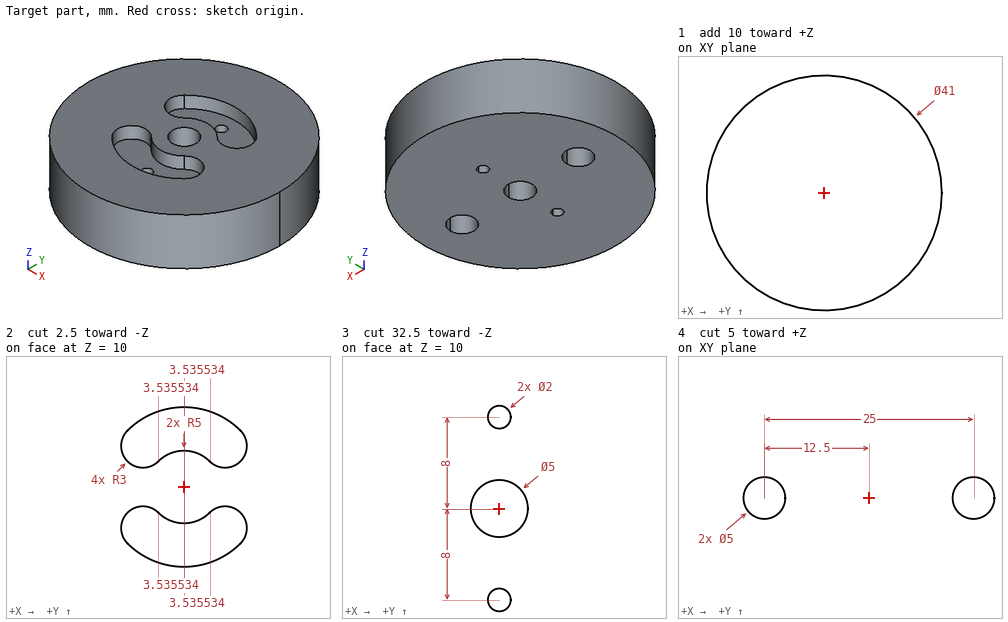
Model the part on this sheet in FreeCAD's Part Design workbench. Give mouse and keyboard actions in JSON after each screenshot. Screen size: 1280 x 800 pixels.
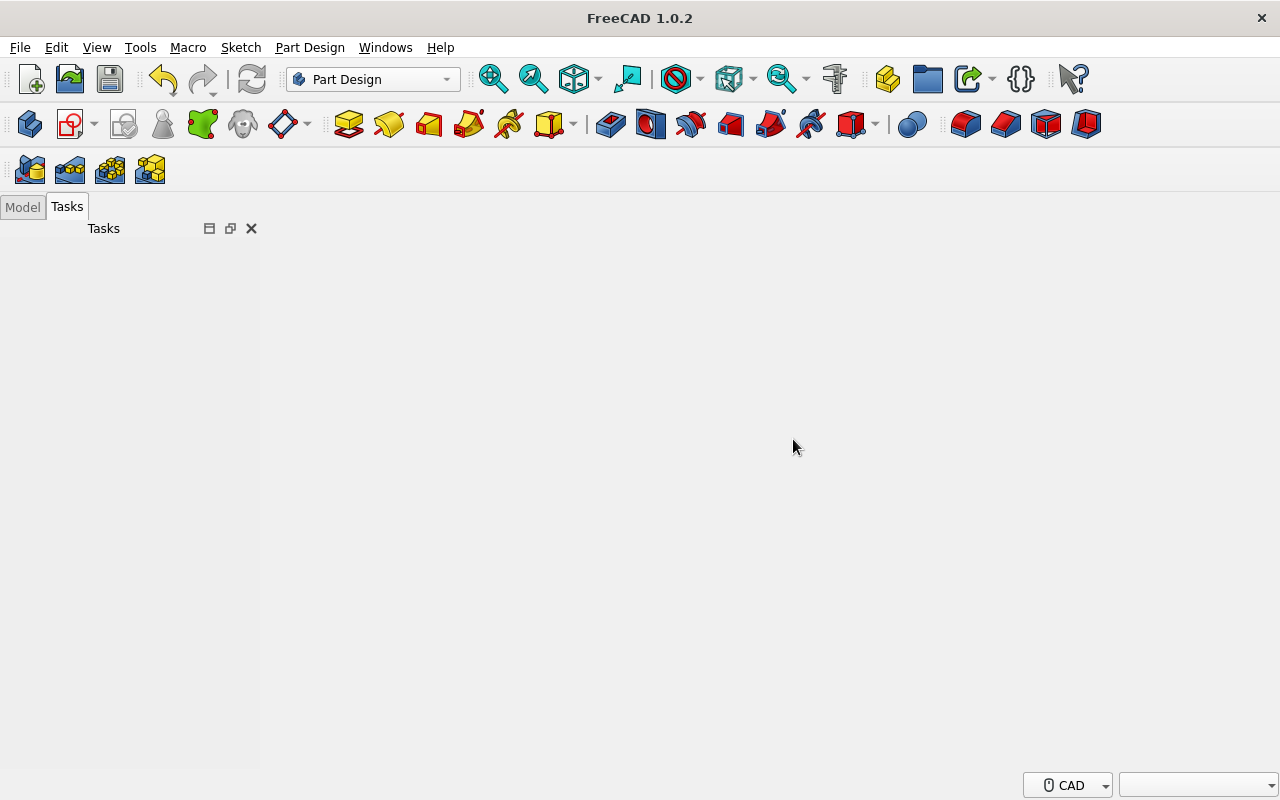
{"action": "key", "text": "ctrl+n"}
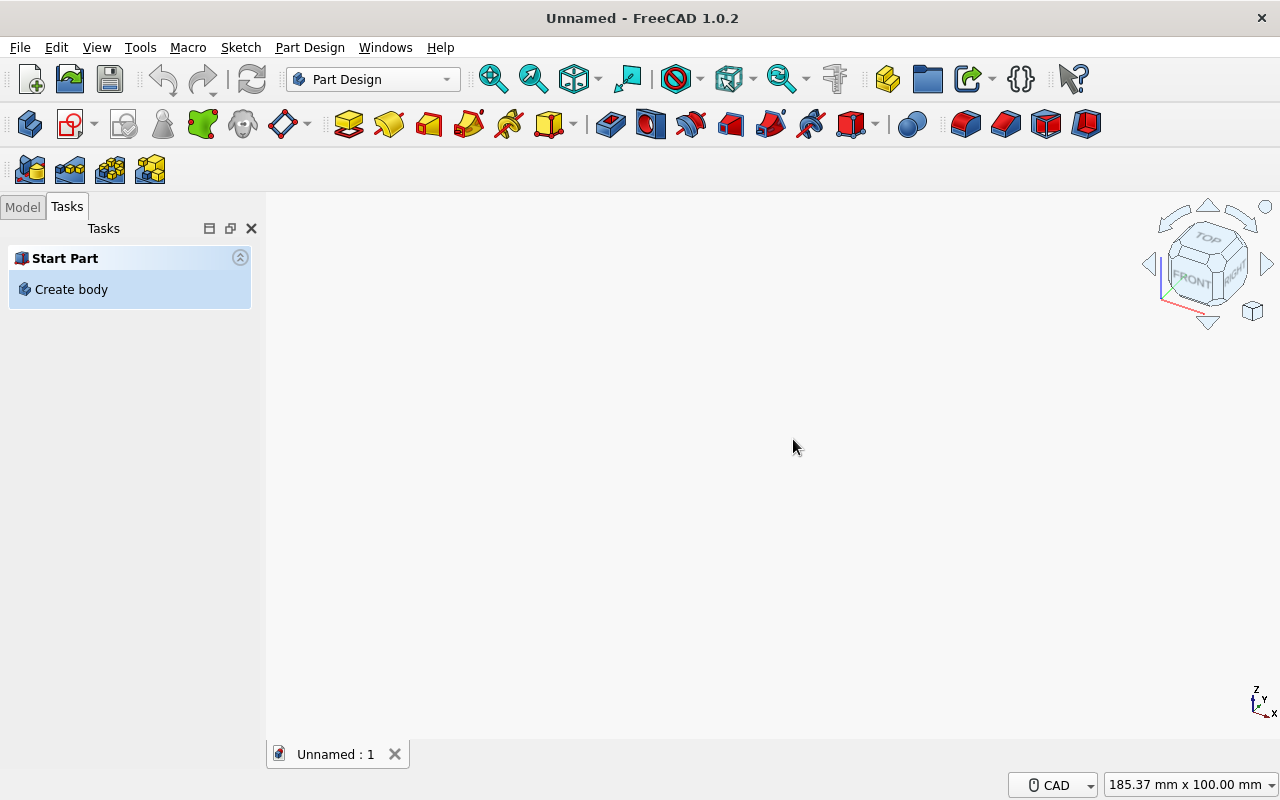
{"action": "left_click", "coordinate": [70, 124]}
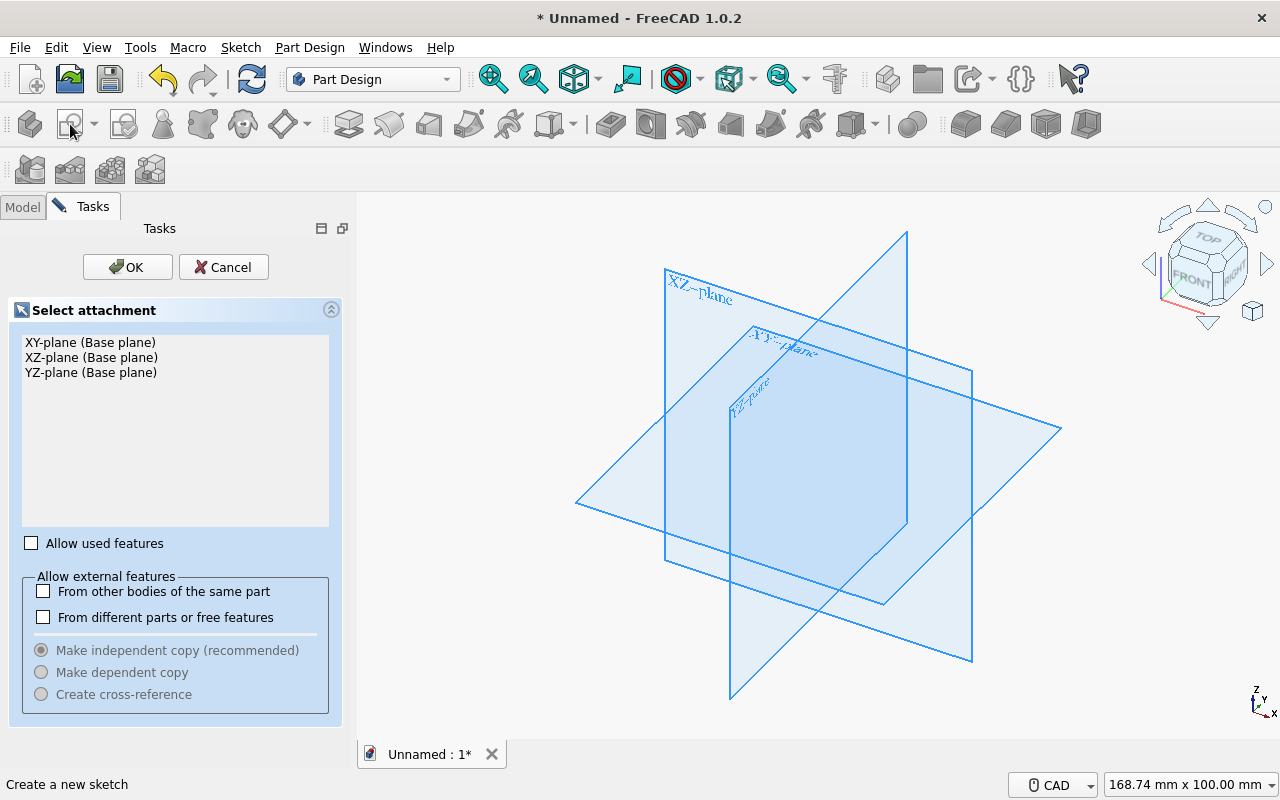
{"action": "left_click", "coordinate": [82, 342]}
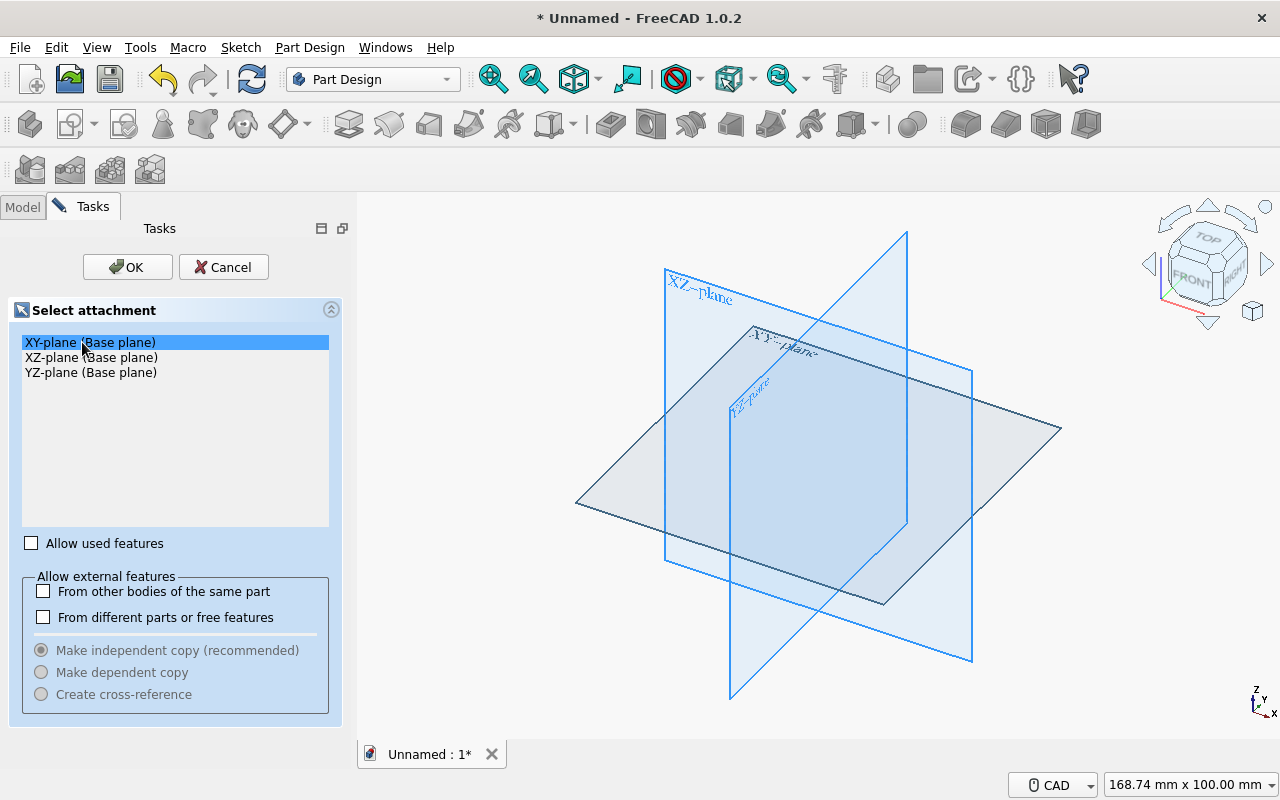
{"action": "left_click", "coordinate": [128, 267]}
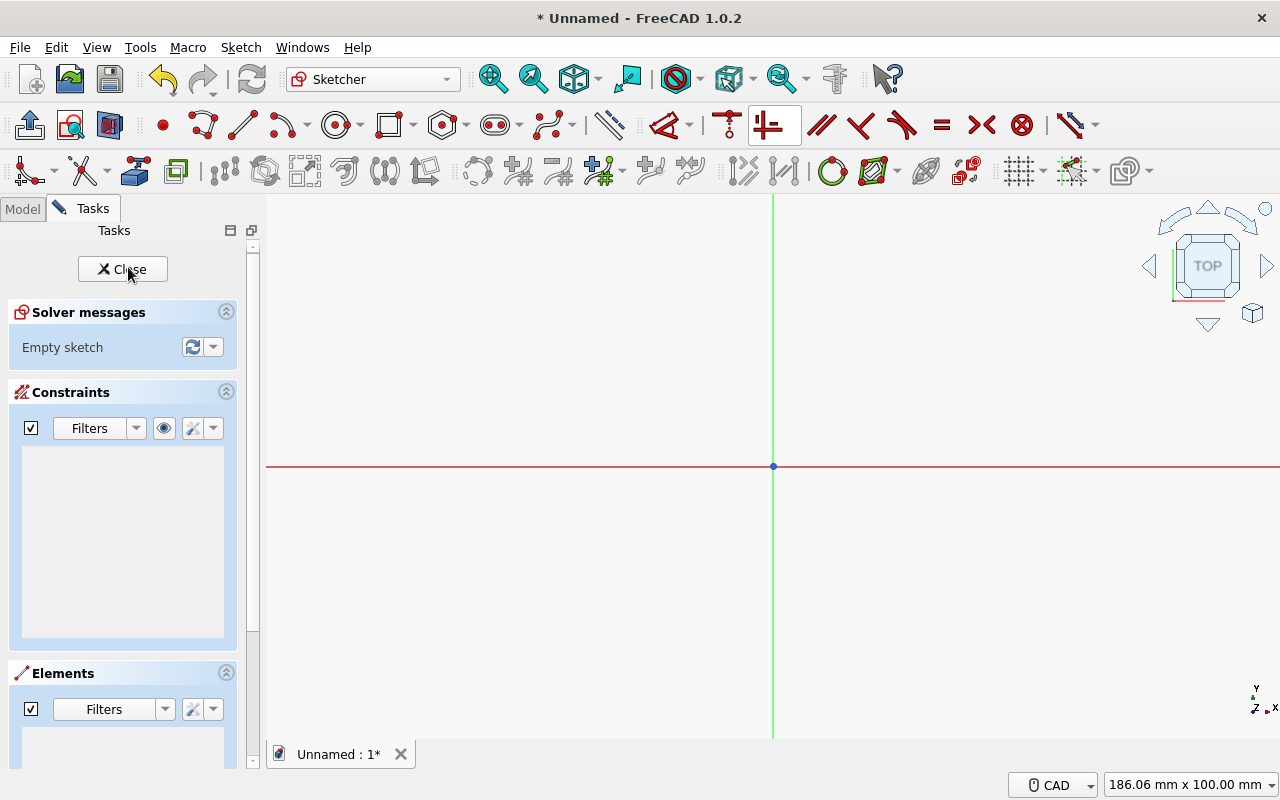
{"action": "scroll", "coordinate": [912, 467], "scroll_direction": "up", "scroll_amount": 2}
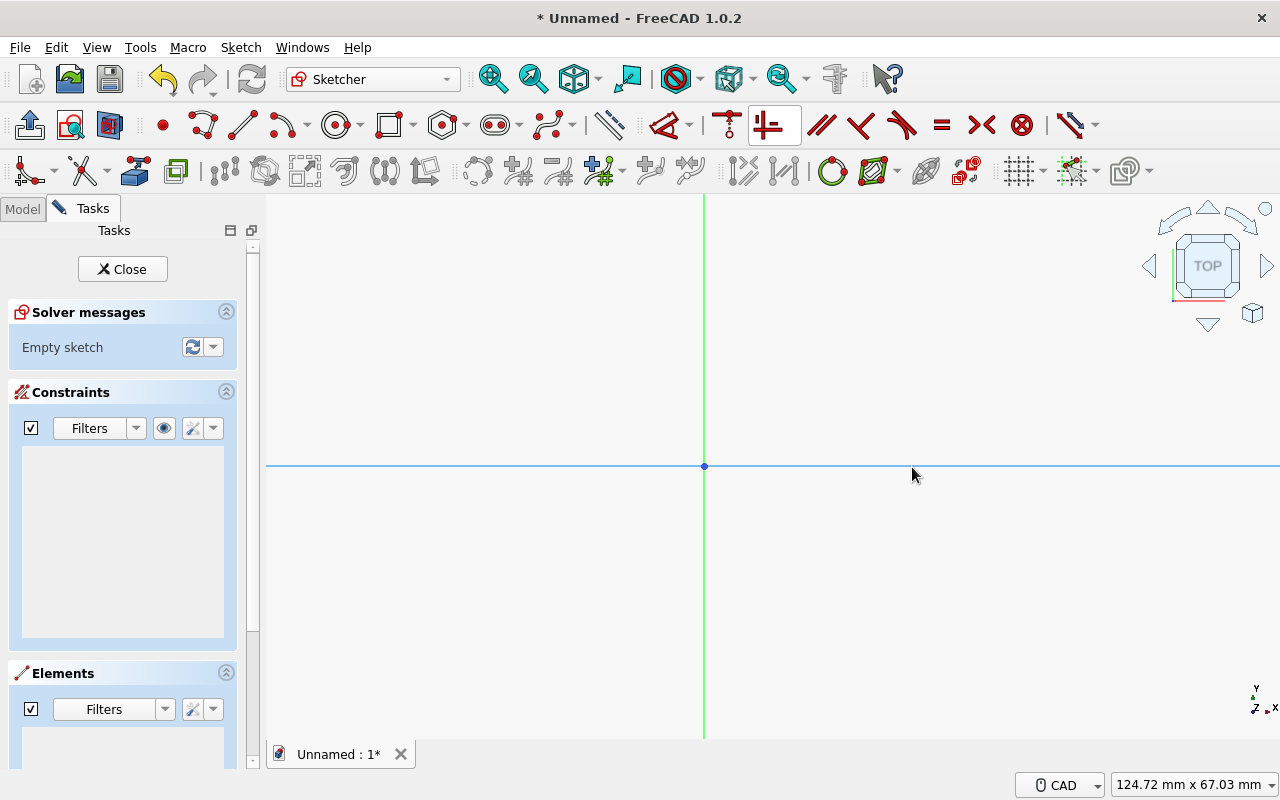
{"action": "key", "text": "g c"}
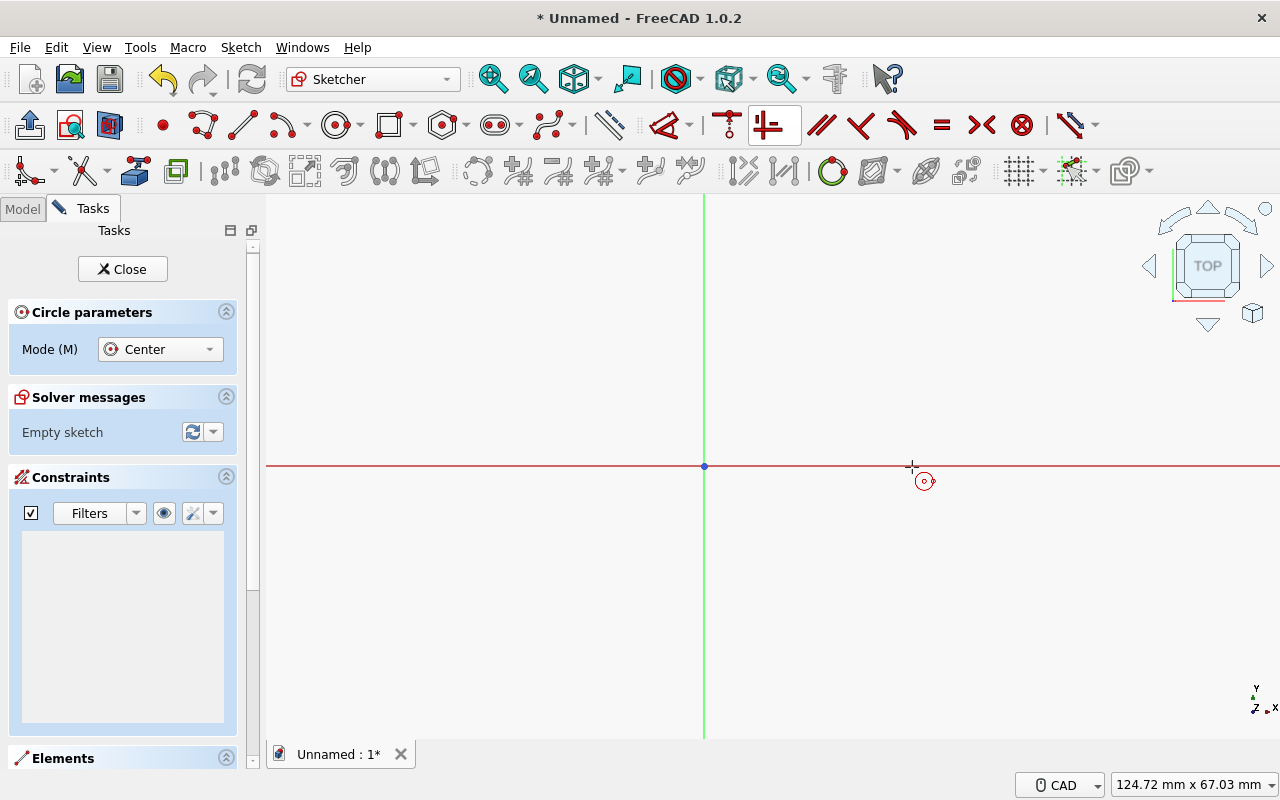
{"action": "left_click", "coordinate": [704, 466]}
{"action": "left_click", "coordinate": [822, 348]}
{"action": "key", "text": "Escape"}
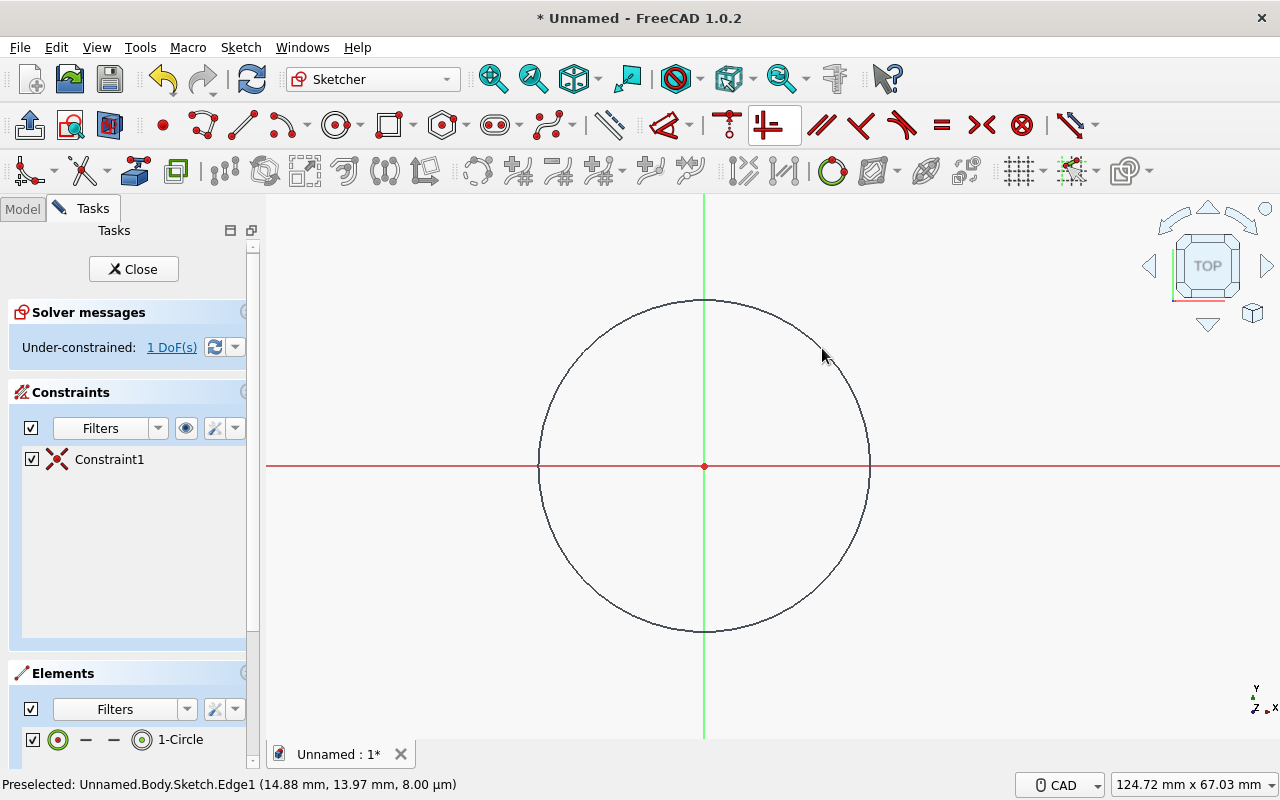
{"action": "key", "text": "d"}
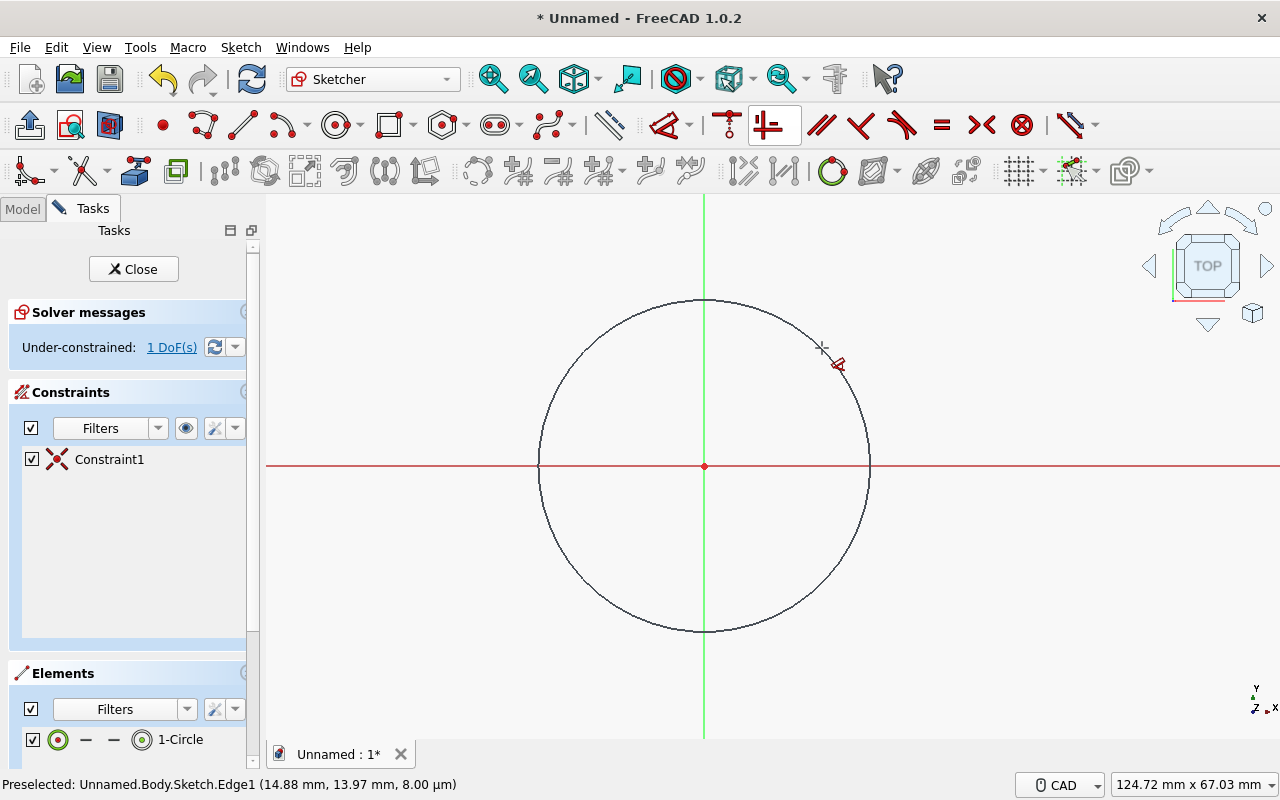
{"action": "left_click", "coordinate": [821, 348]}
{"action": "left_click", "coordinate": [843, 325]}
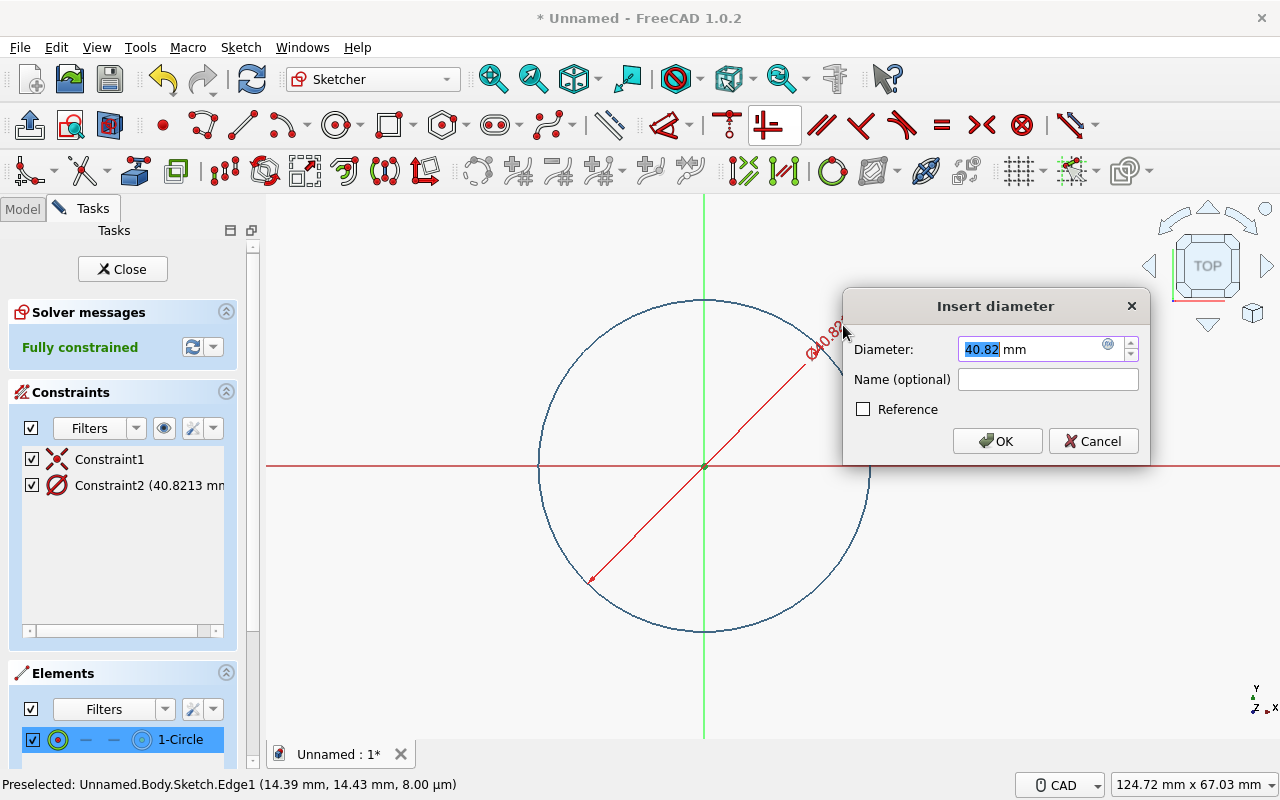
{"action": "type", "text": "41"}
{"action": "key", "text": "Return"}
{"action": "key", "text": "Escape"}